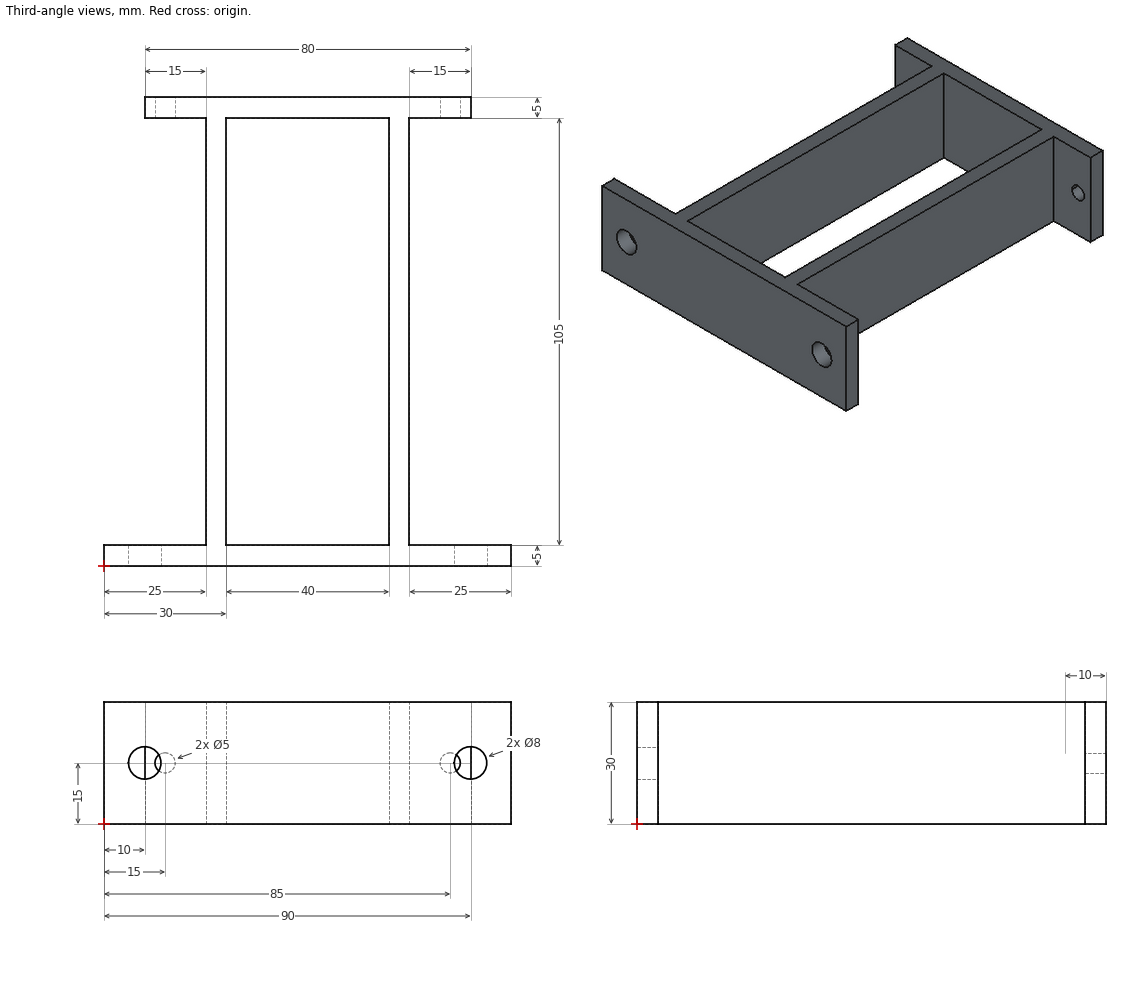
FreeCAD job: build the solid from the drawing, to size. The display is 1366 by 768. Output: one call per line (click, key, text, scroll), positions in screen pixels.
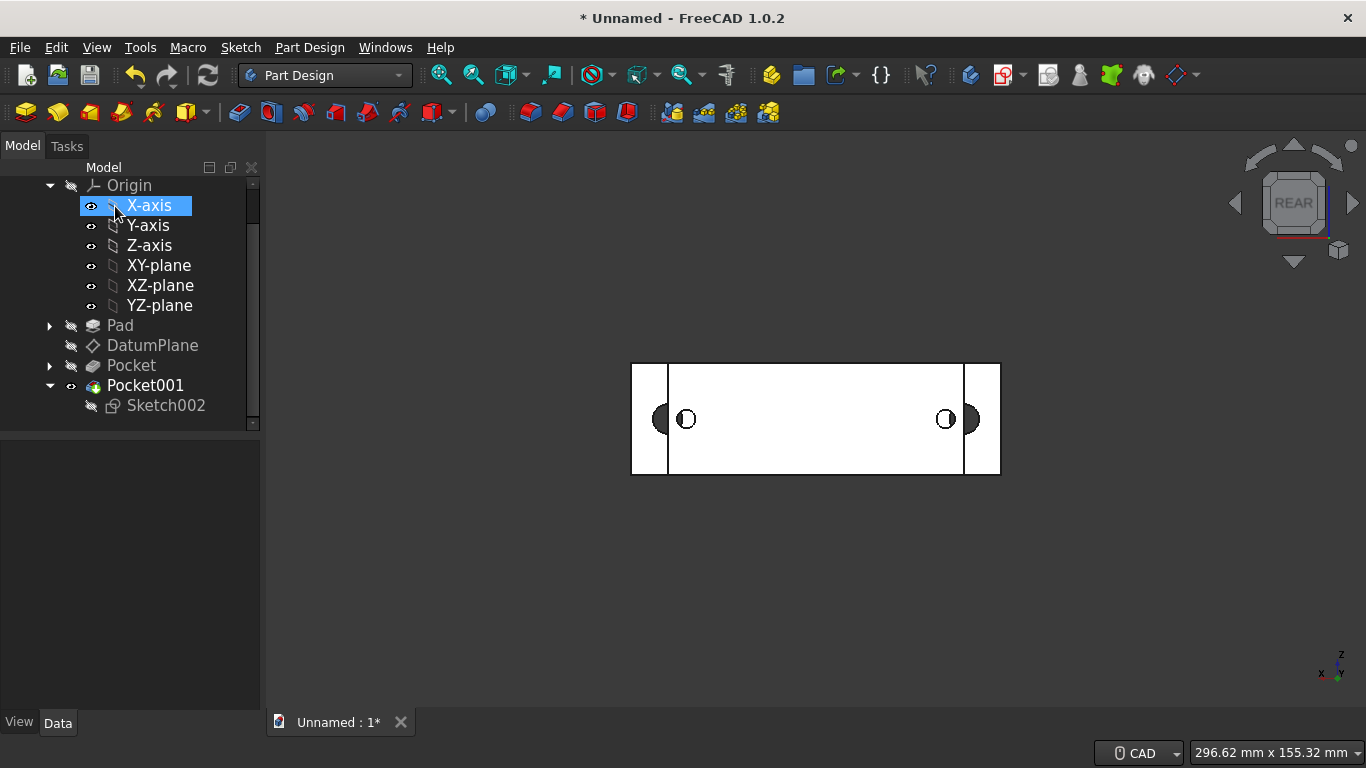
key(0)